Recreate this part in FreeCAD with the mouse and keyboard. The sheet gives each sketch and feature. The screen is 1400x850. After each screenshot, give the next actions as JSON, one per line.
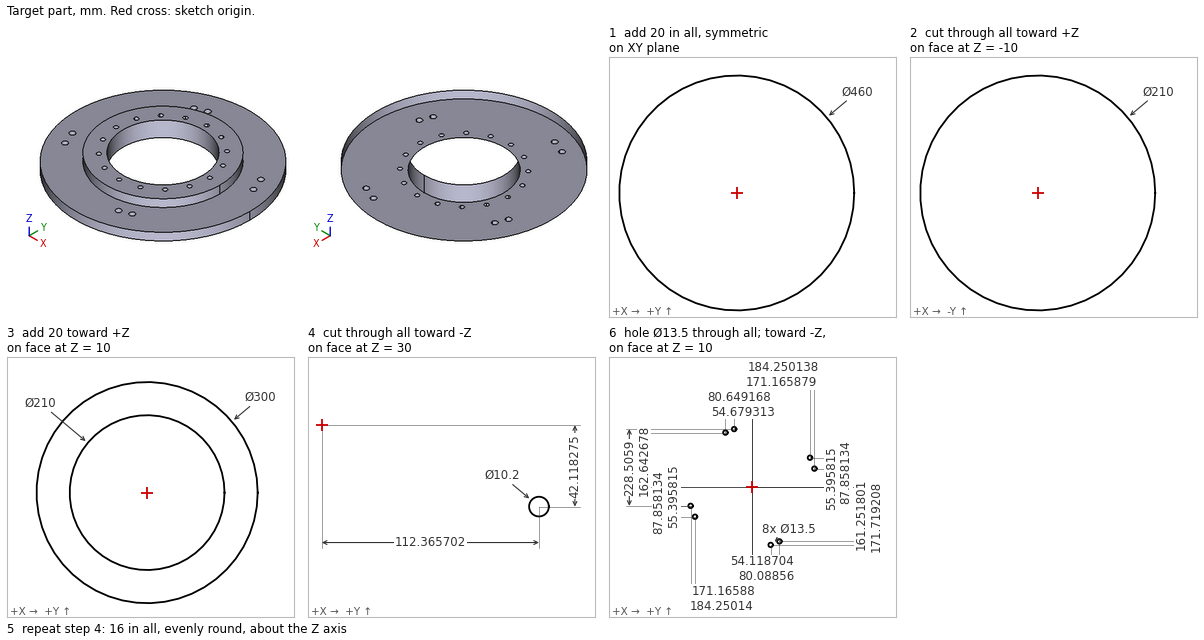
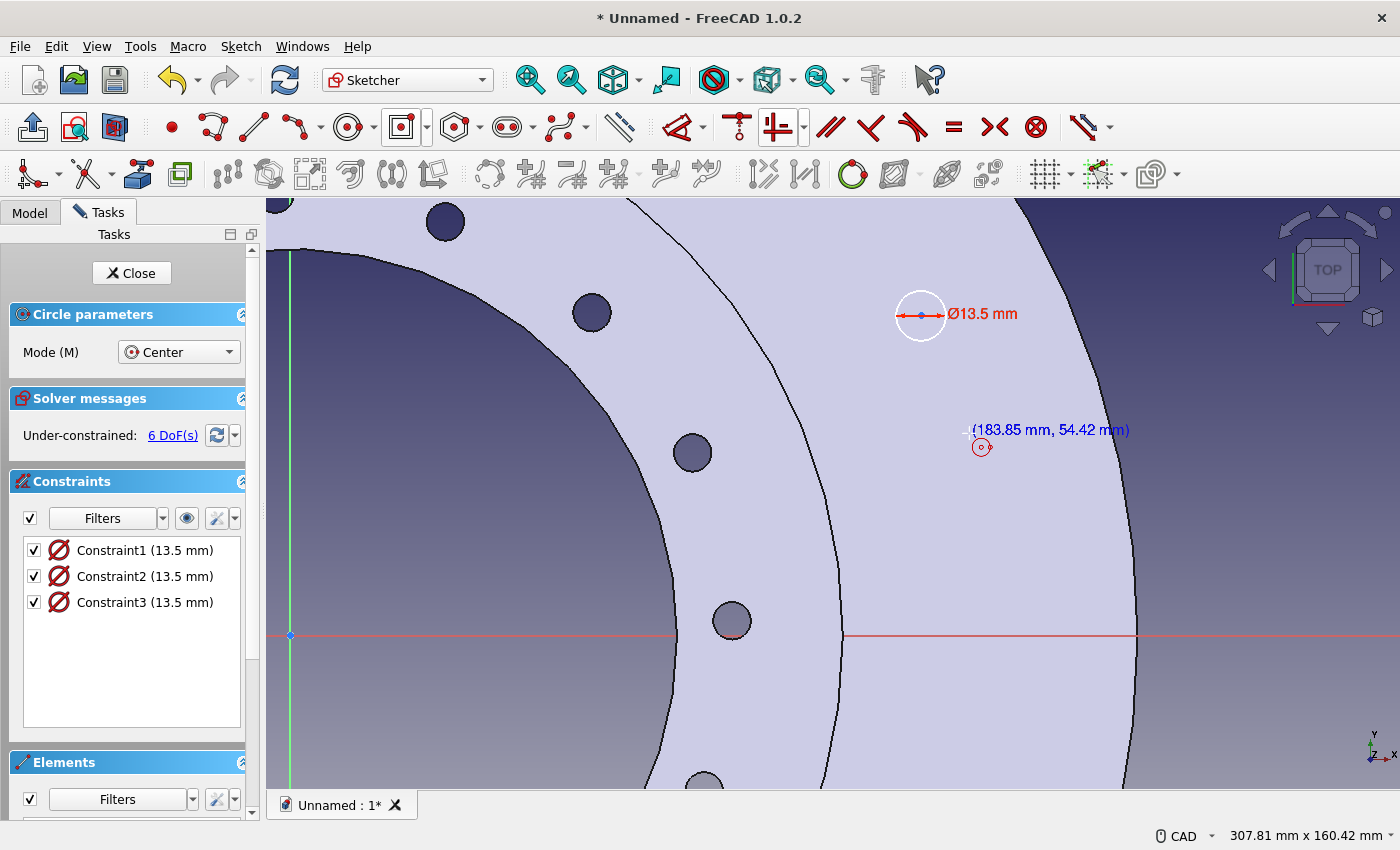
{"action": "scroll", "coordinate": [969, 433], "scroll_direction": "down", "scroll_amount": 6}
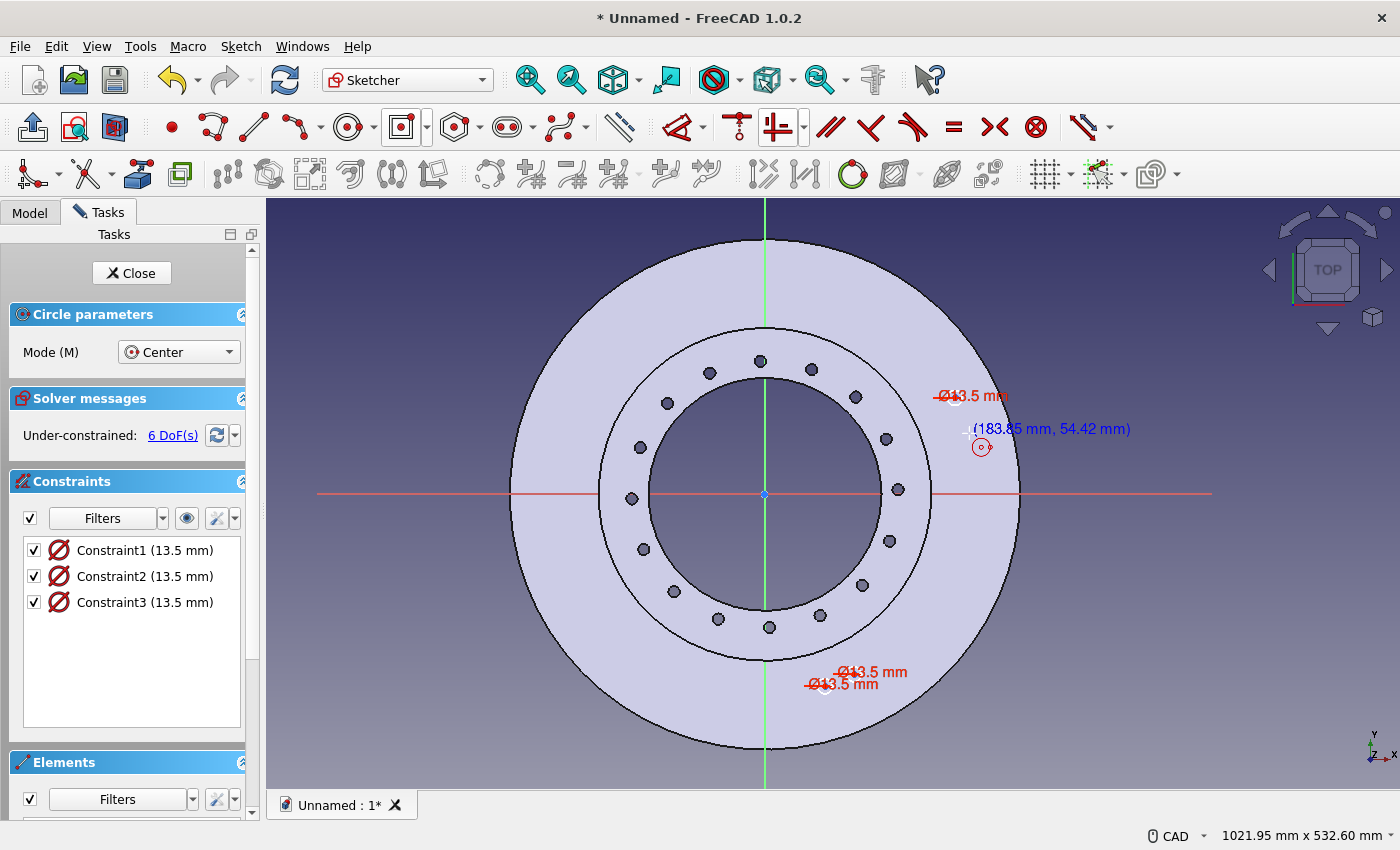
{"action": "left_click", "coordinate": [969, 433]}
{"action": "mouse_move", "coordinate": [975, 428]}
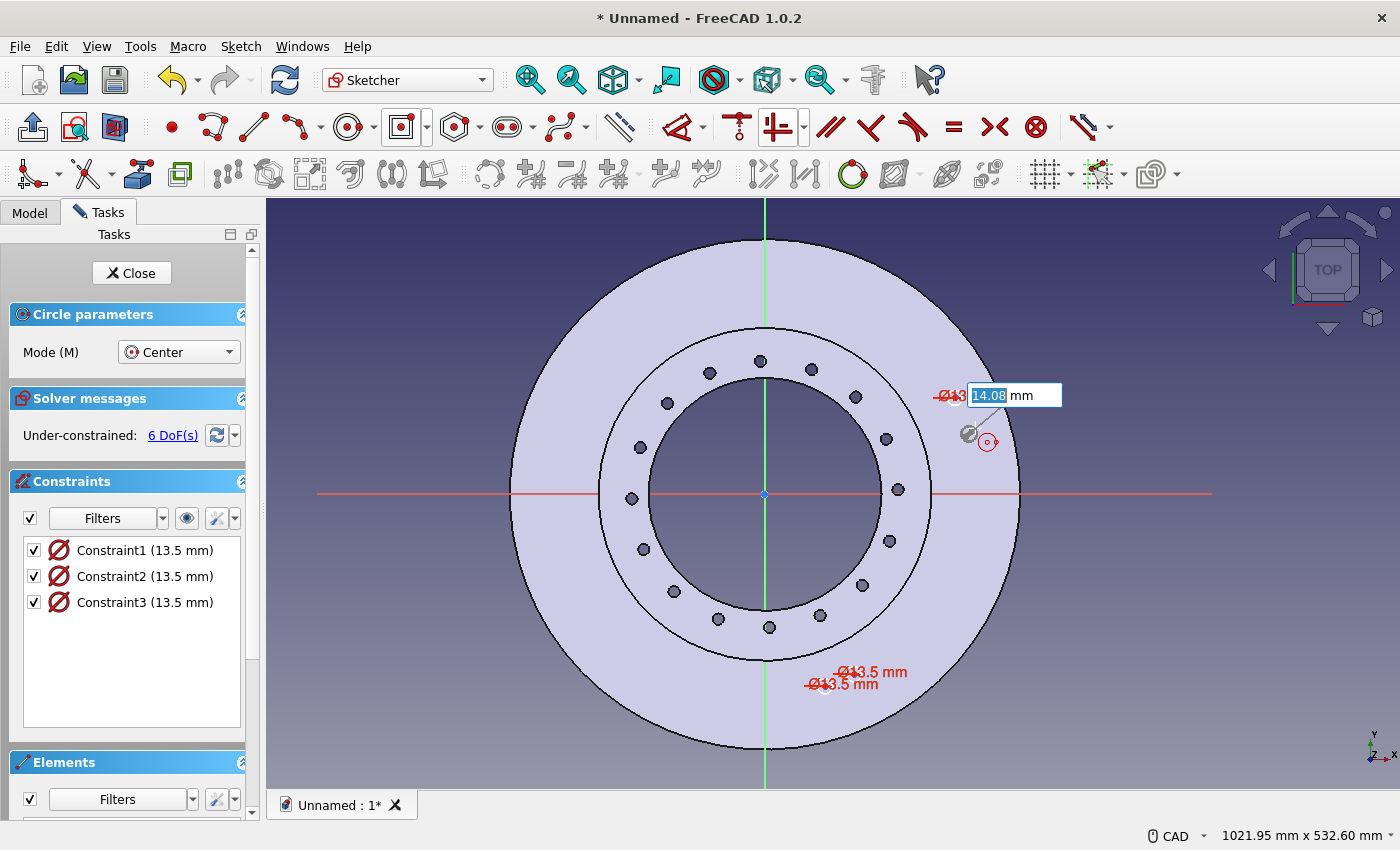
{"action": "type", "text": "13.5"}
{"action": "key", "text": "Return"}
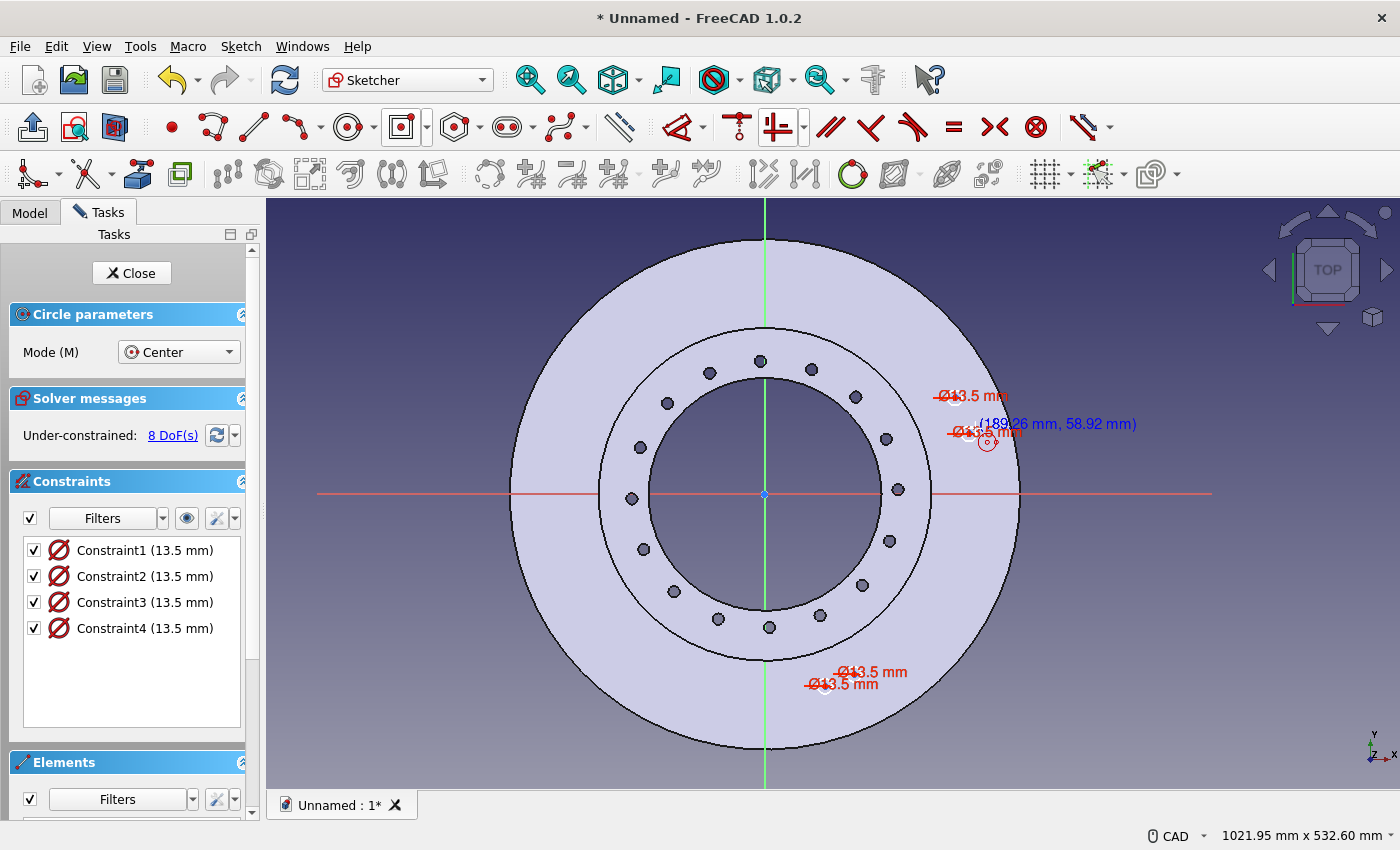
{"action": "scroll", "coordinate": [575, 592], "scroll_direction": "up", "scroll_amount": 6}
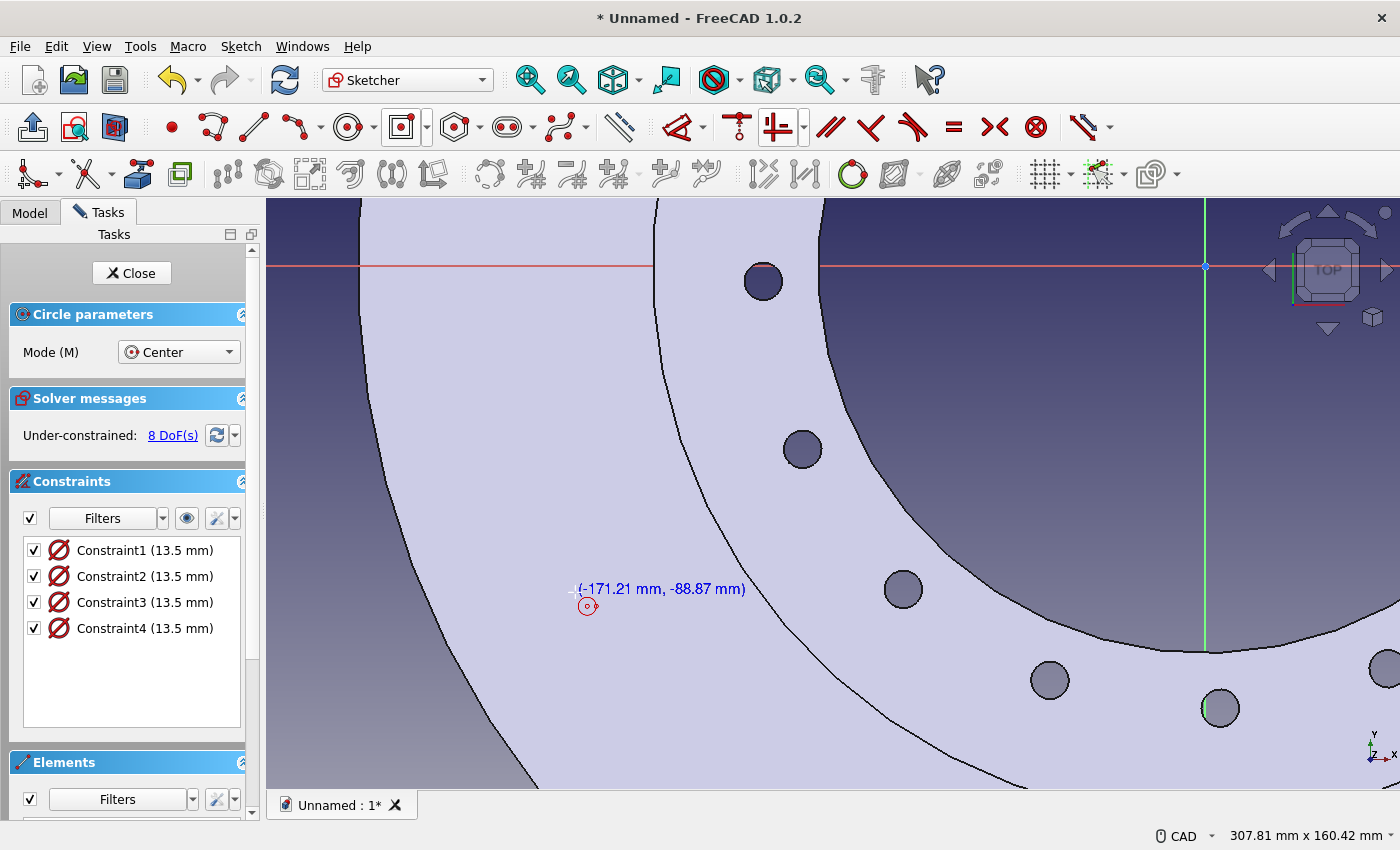
{"action": "scroll", "coordinate": [575, 593], "scroll_direction": "down", "scroll_amount": 6}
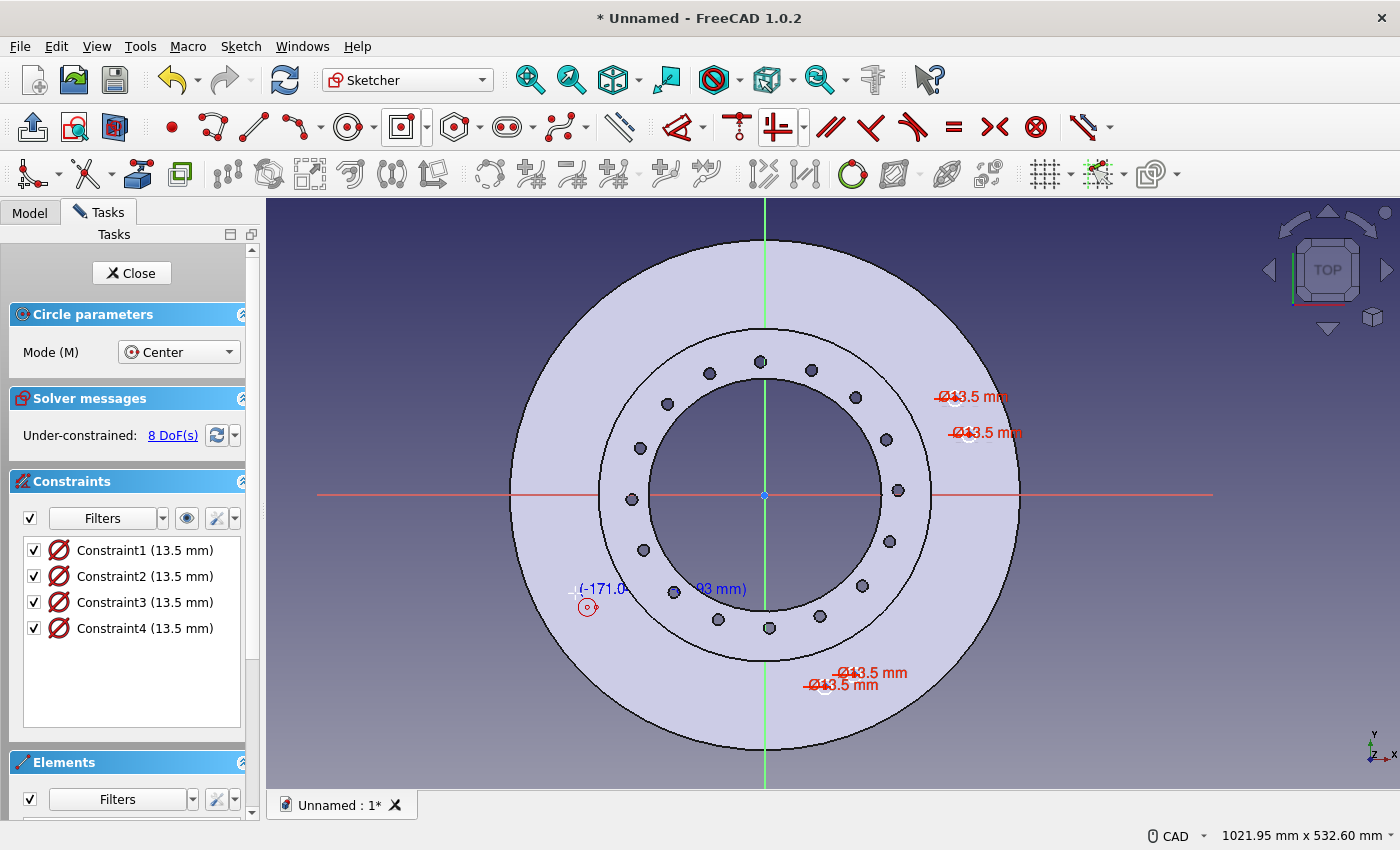
{"action": "left_click", "coordinate": [575, 593]}
{"action": "mouse_move", "coordinate": [580, 587]}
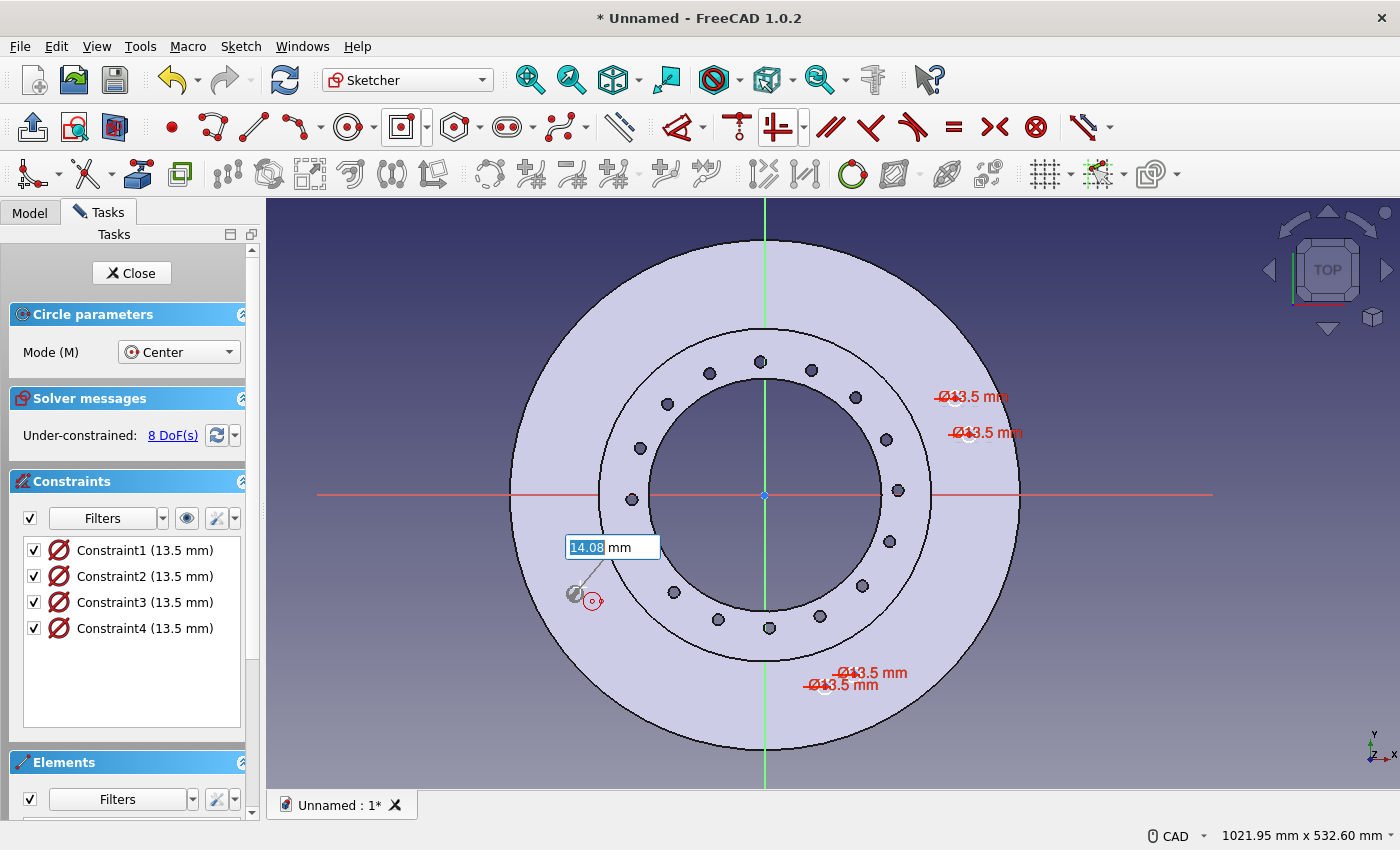
{"action": "type", "text": "13.5"}
{"action": "key", "text": "Return"}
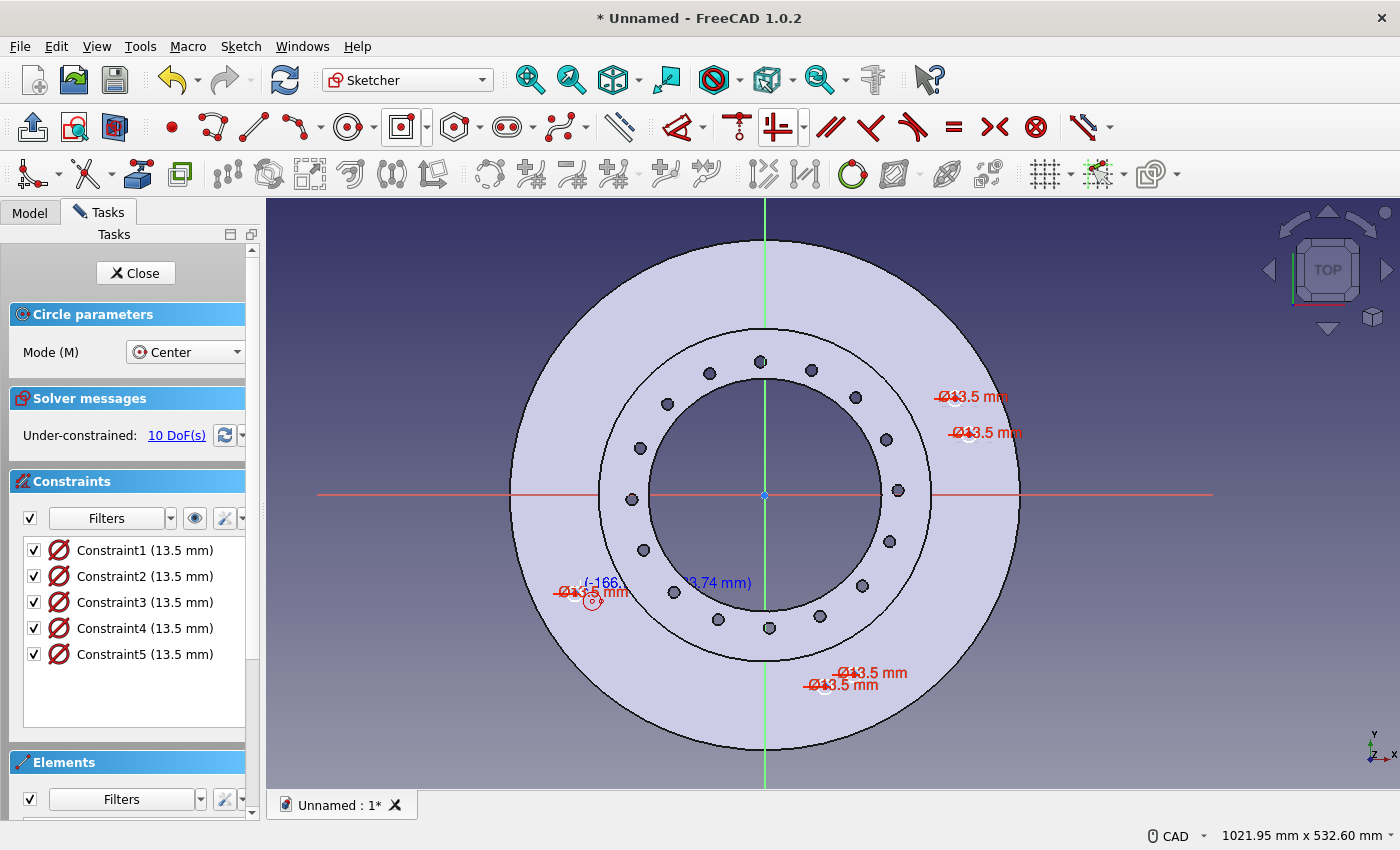
{"action": "scroll", "coordinate": [561, 557], "scroll_direction": "up", "scroll_amount": 6}